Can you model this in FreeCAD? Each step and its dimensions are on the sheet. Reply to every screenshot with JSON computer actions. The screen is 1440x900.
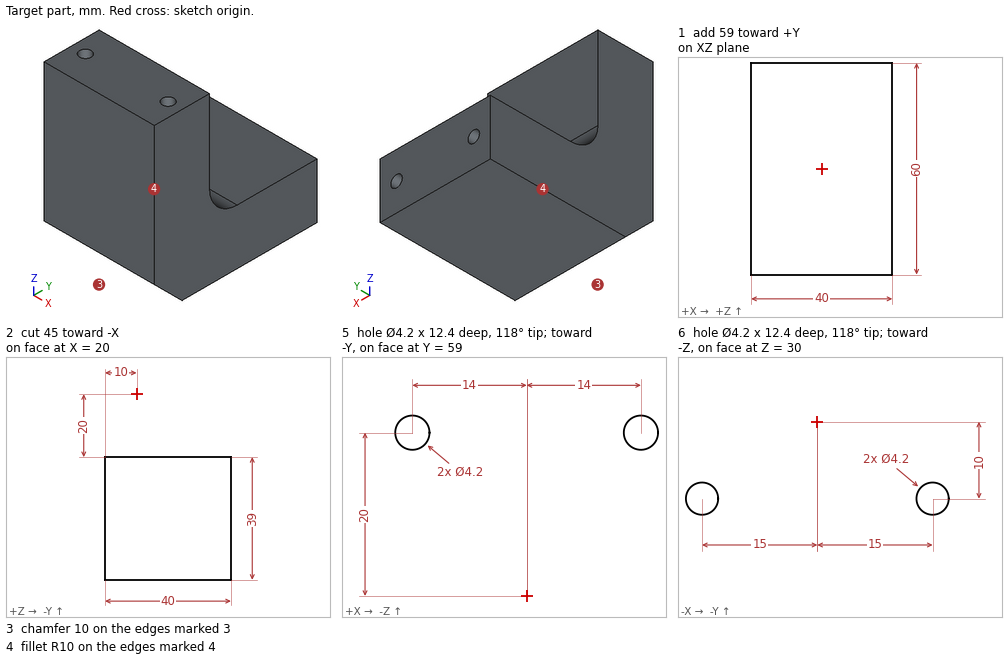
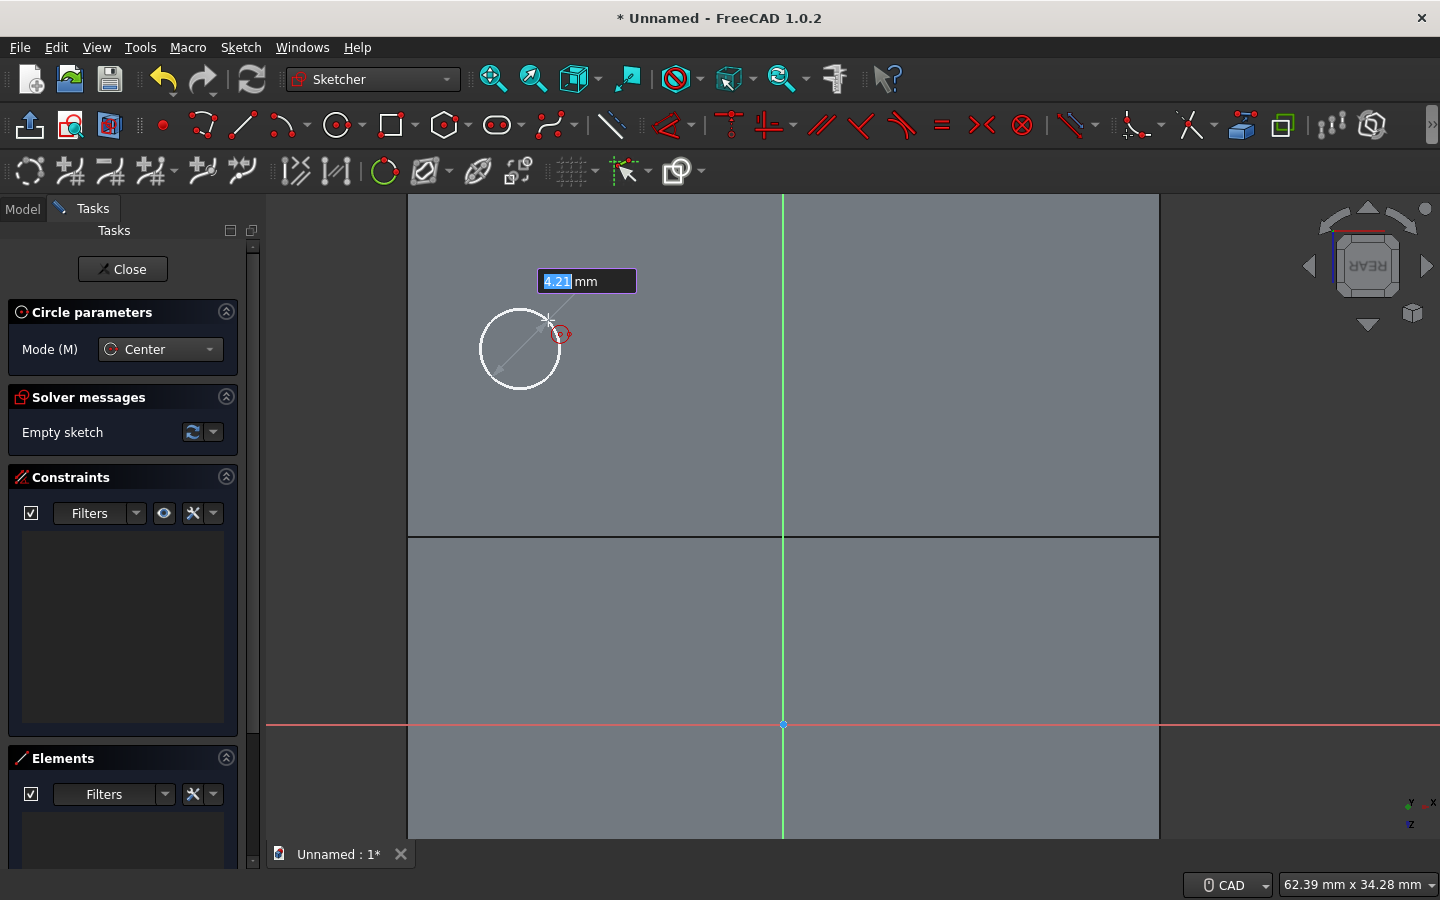
{"action": "type", "text": "4.2"}
{"action": "key", "text": "Return"}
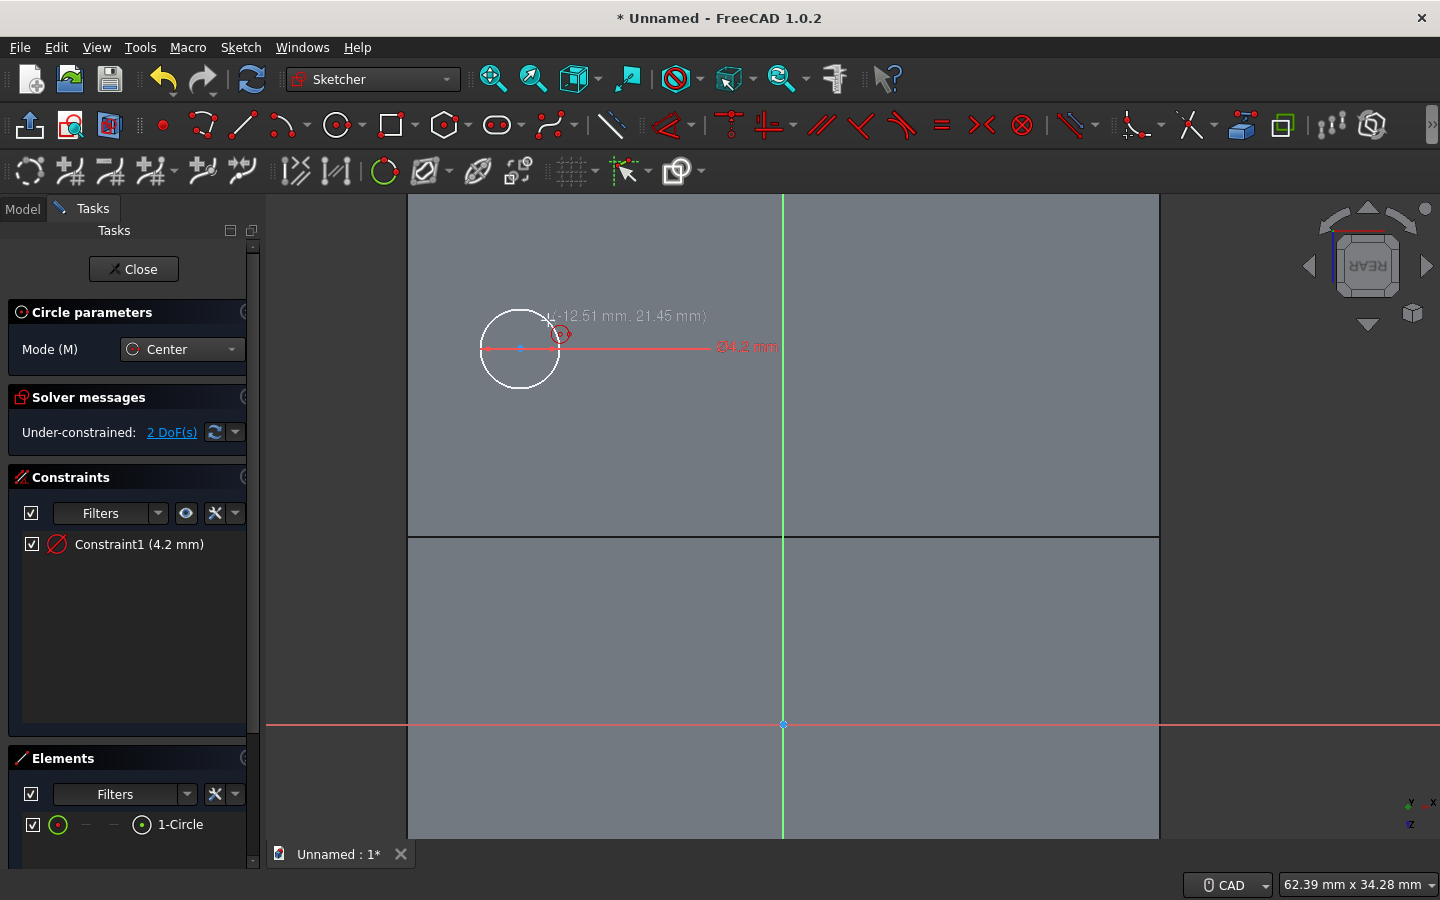
{"action": "left_click", "coordinate": [1047, 348]}
{"action": "mouse_move", "coordinate": [1075, 320]}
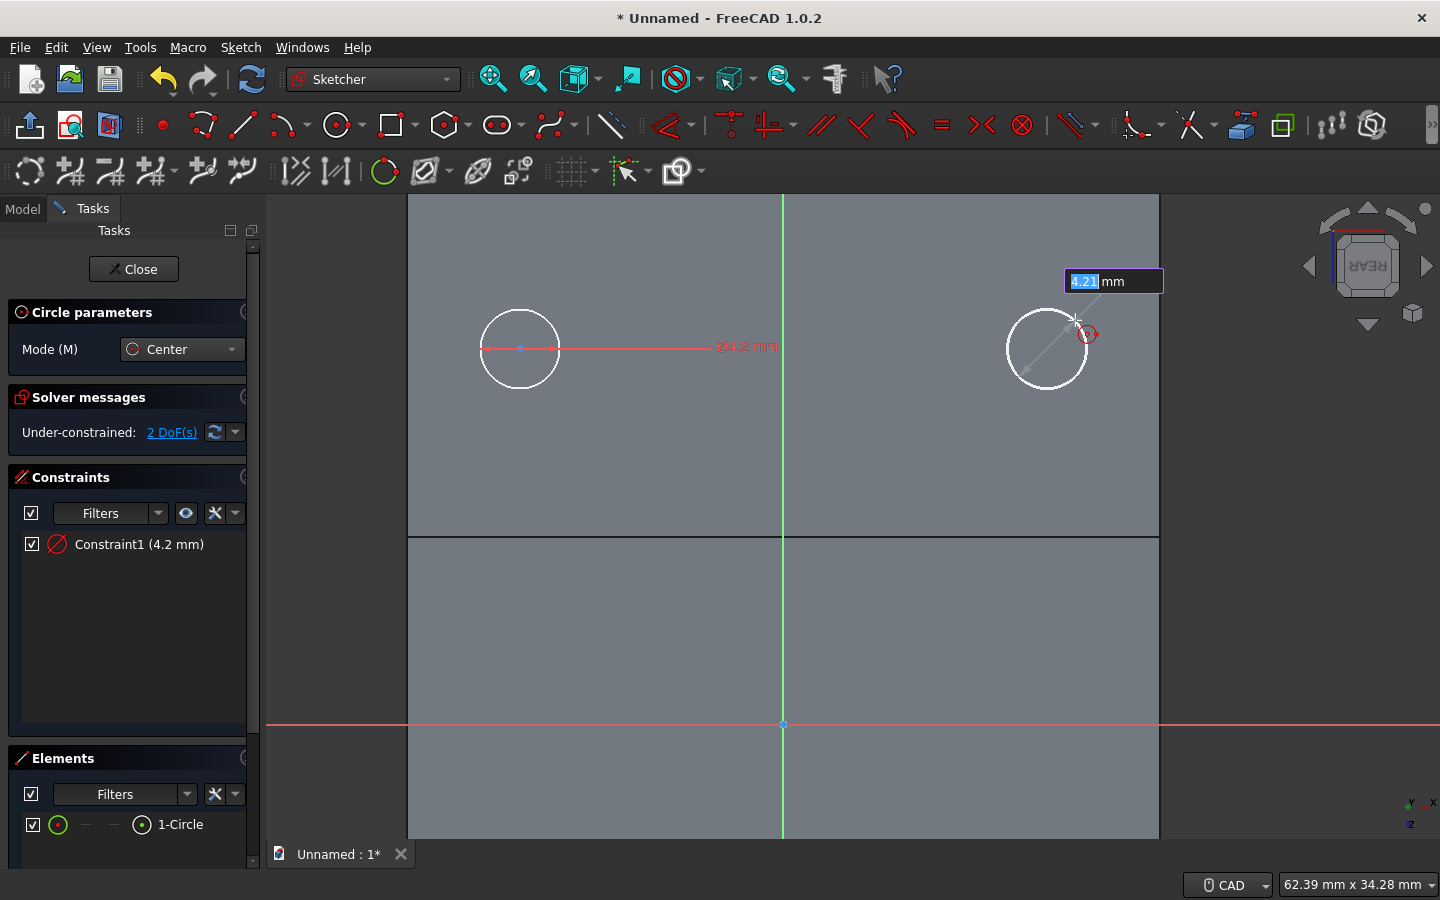
{"action": "type", "text": "4.2"}
{"action": "key", "text": "Return"}
{"action": "key", "text": "Escape"}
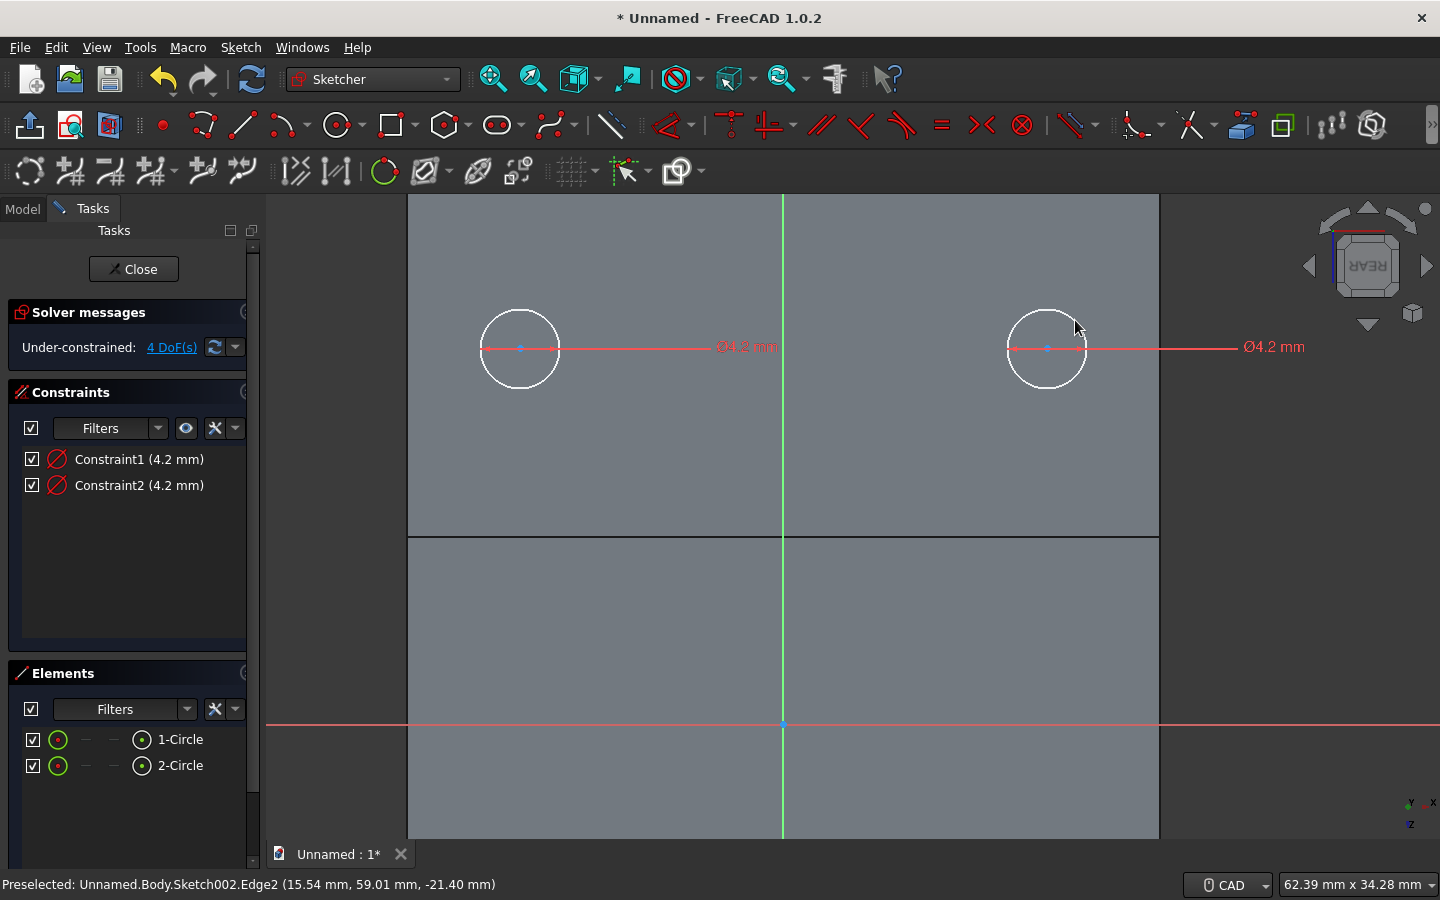
{"action": "left_click", "coordinate": [520, 349]}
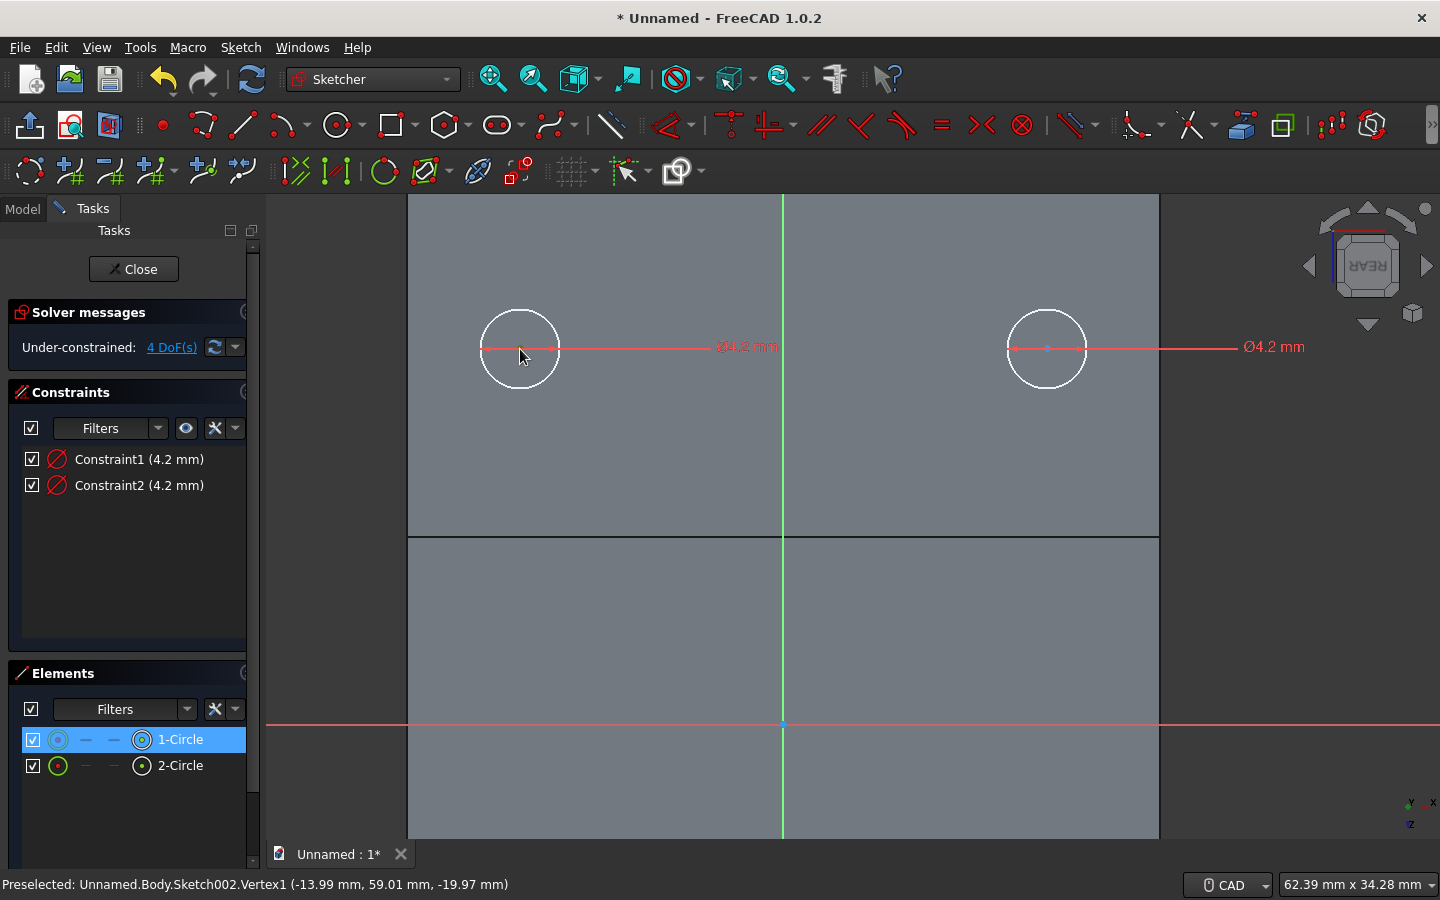
{"action": "left_click", "coordinate": [1047, 349]}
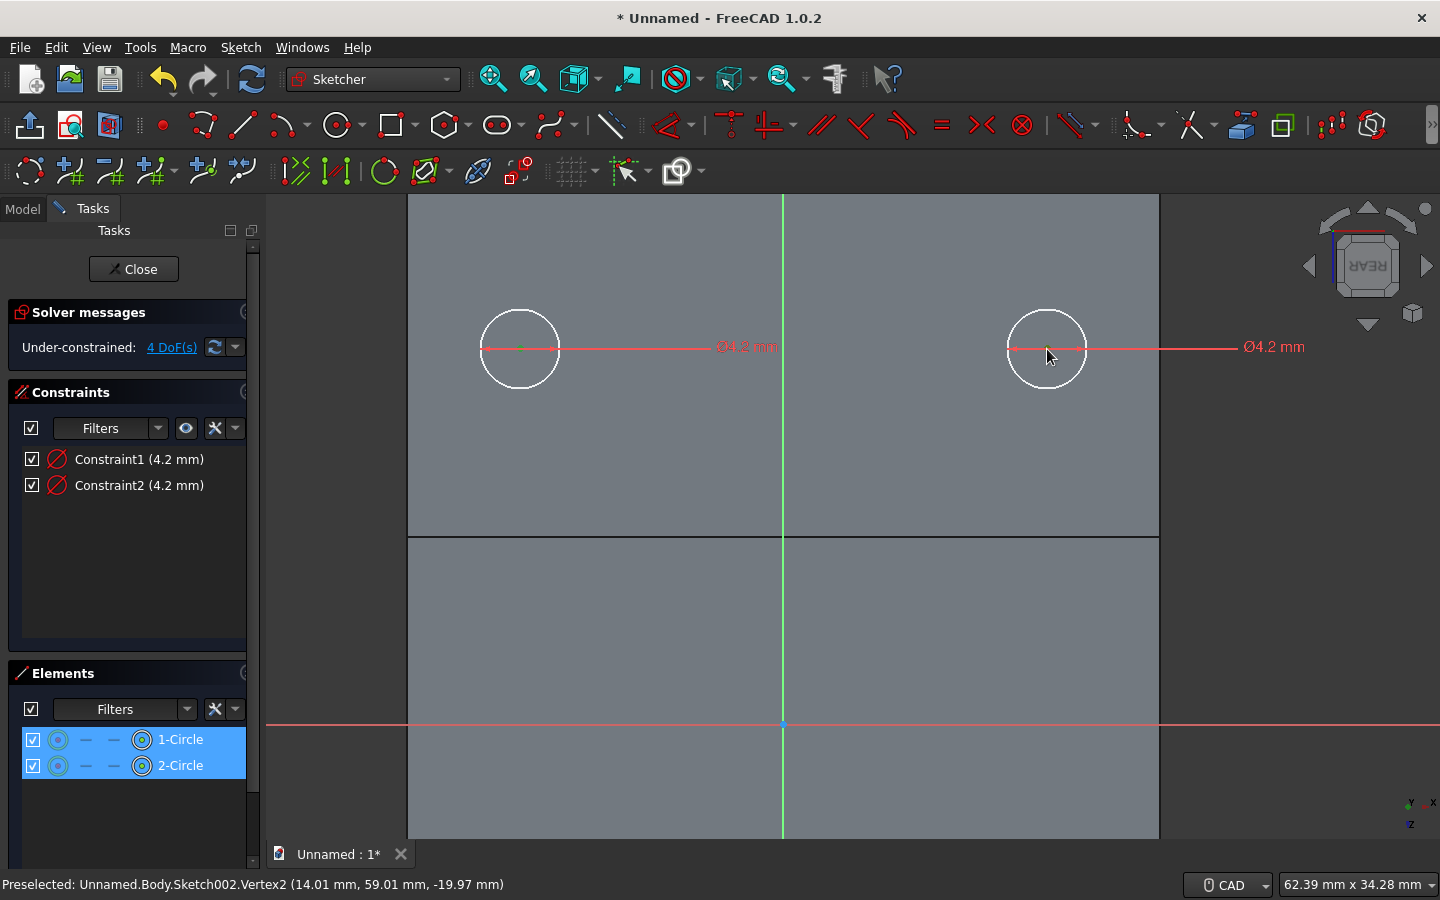
{"action": "key", "text": "h"}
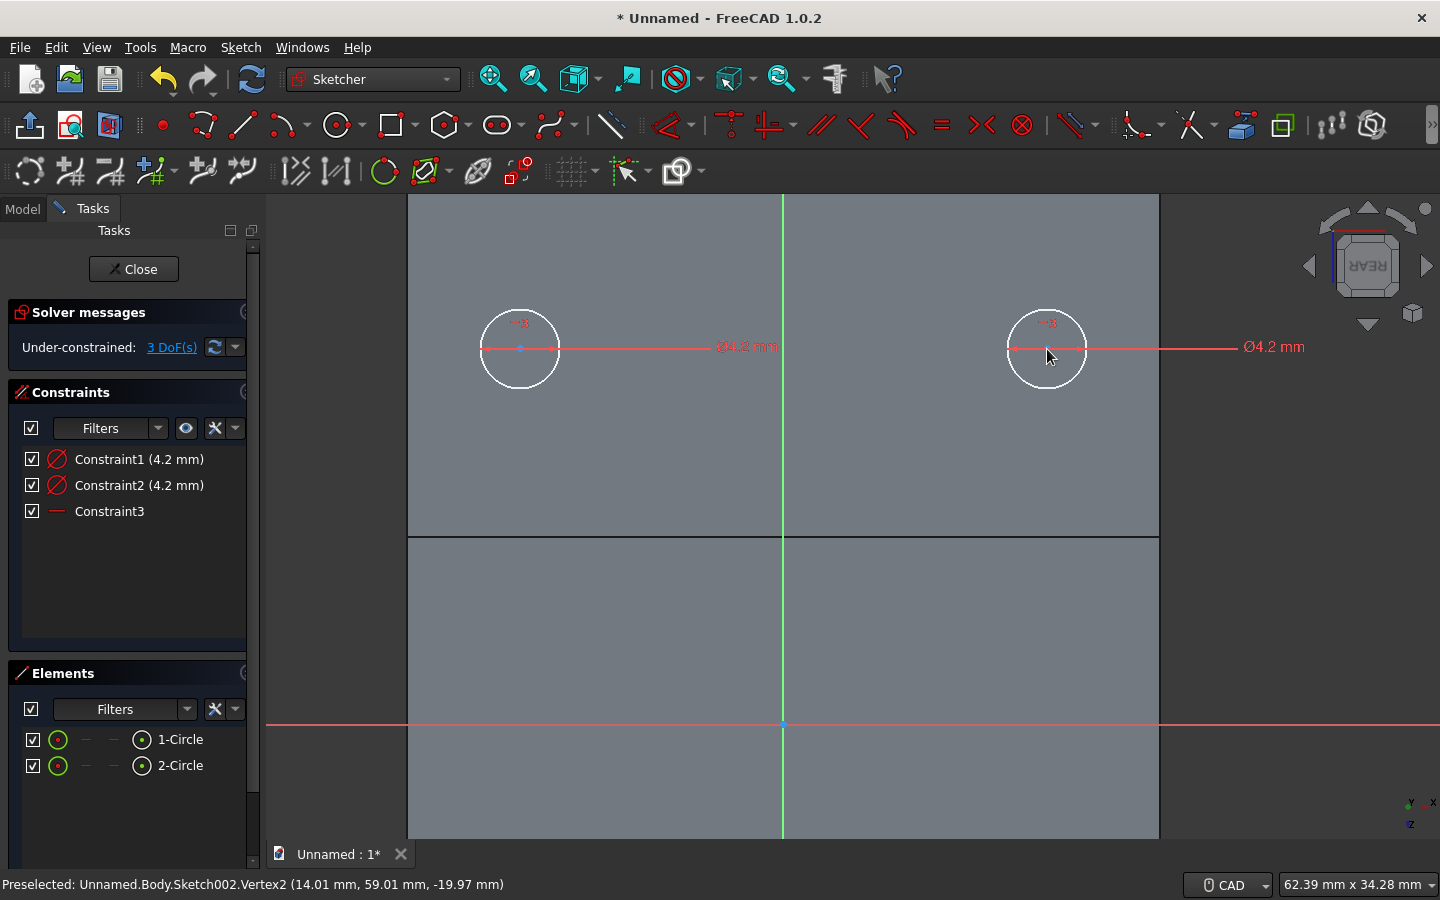
{"action": "left_click", "coordinate": [666, 126]}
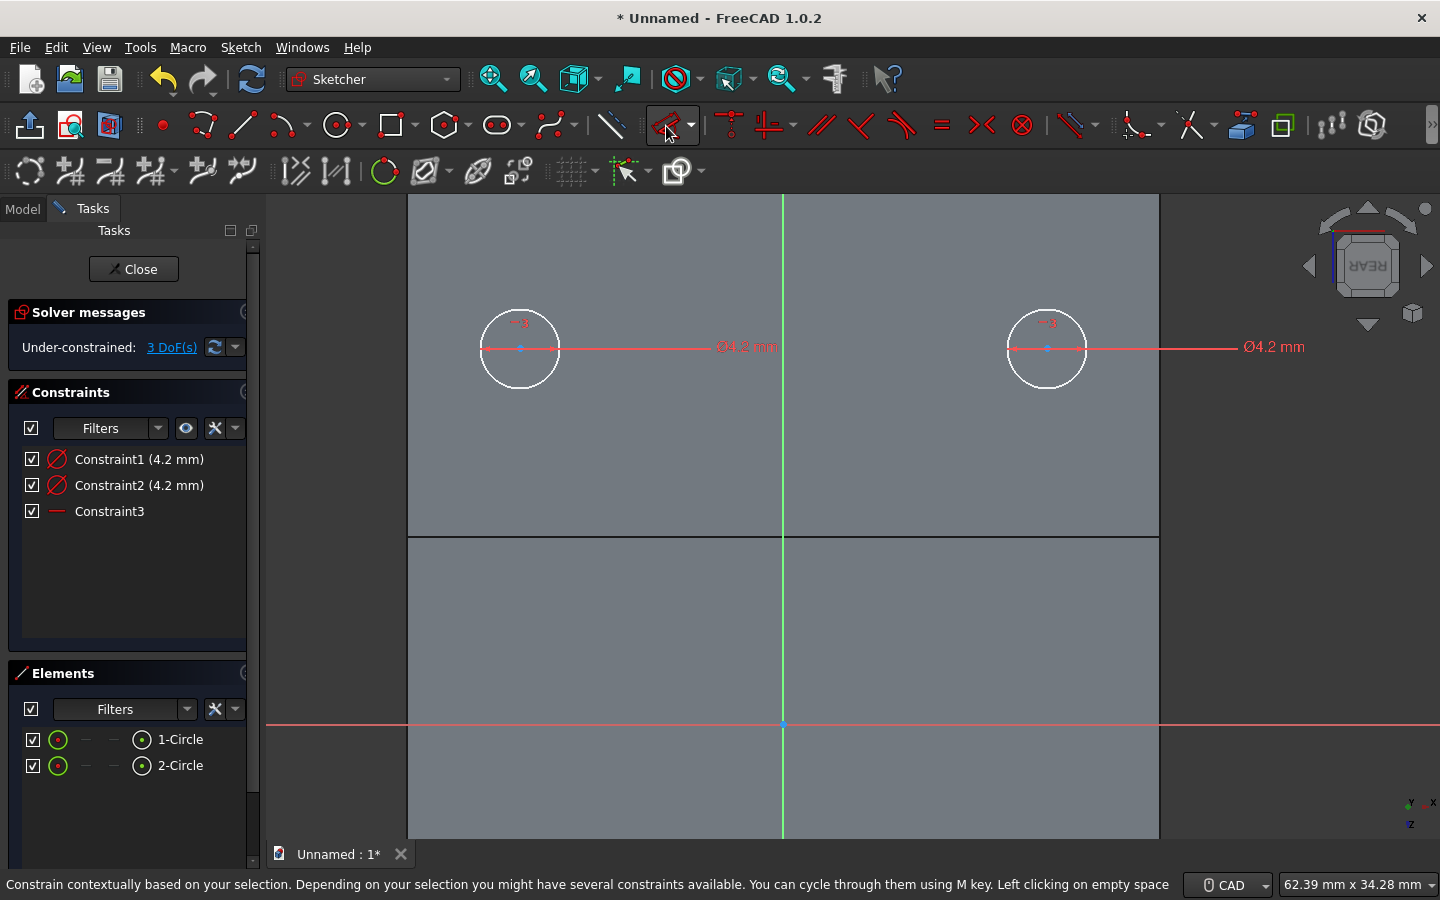
{"action": "left_click", "coordinate": [520, 349]}
{"action": "left_click", "coordinate": [652, 759]}